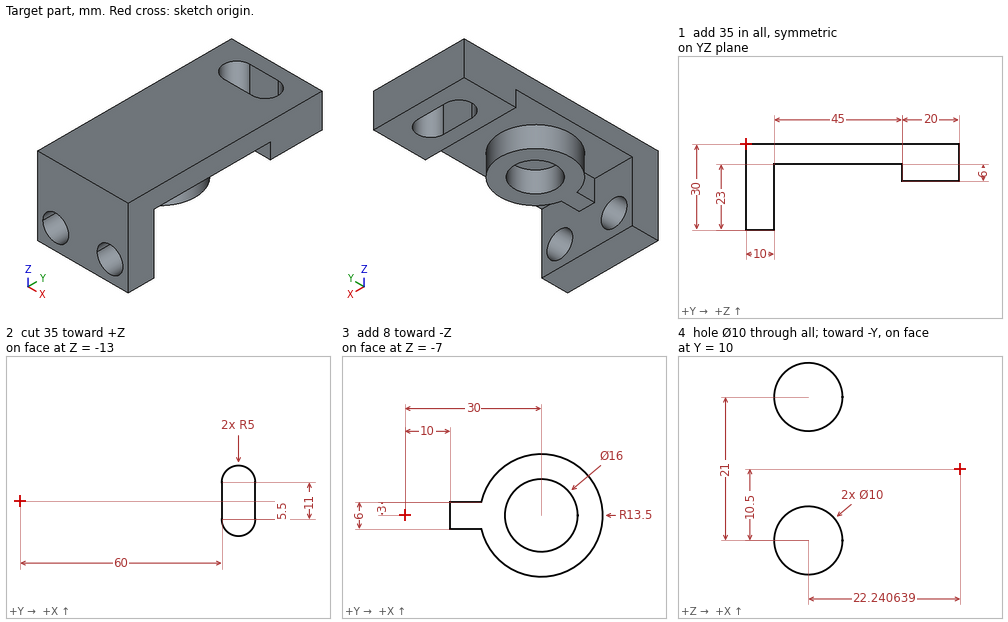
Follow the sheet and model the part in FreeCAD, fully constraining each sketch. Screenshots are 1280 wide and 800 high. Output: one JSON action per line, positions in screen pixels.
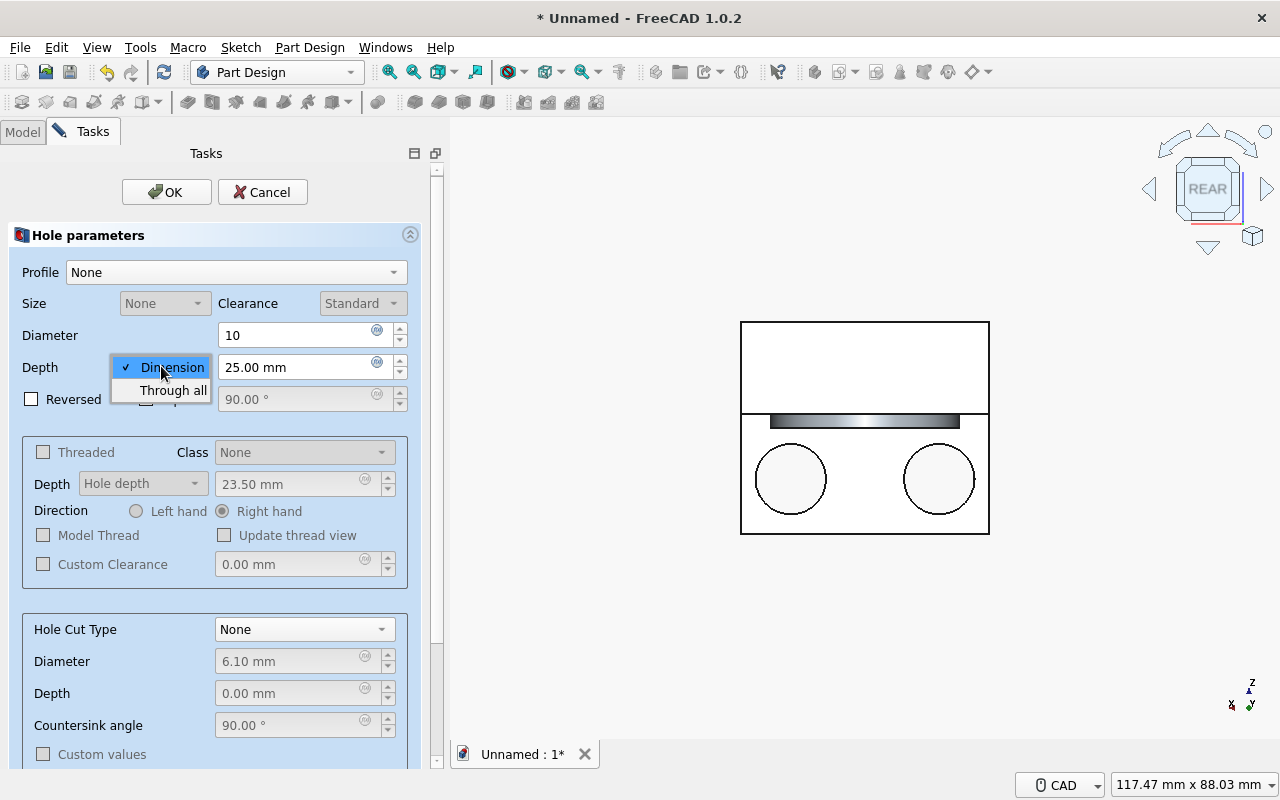
{"action": "left_click", "coordinate": [160, 390]}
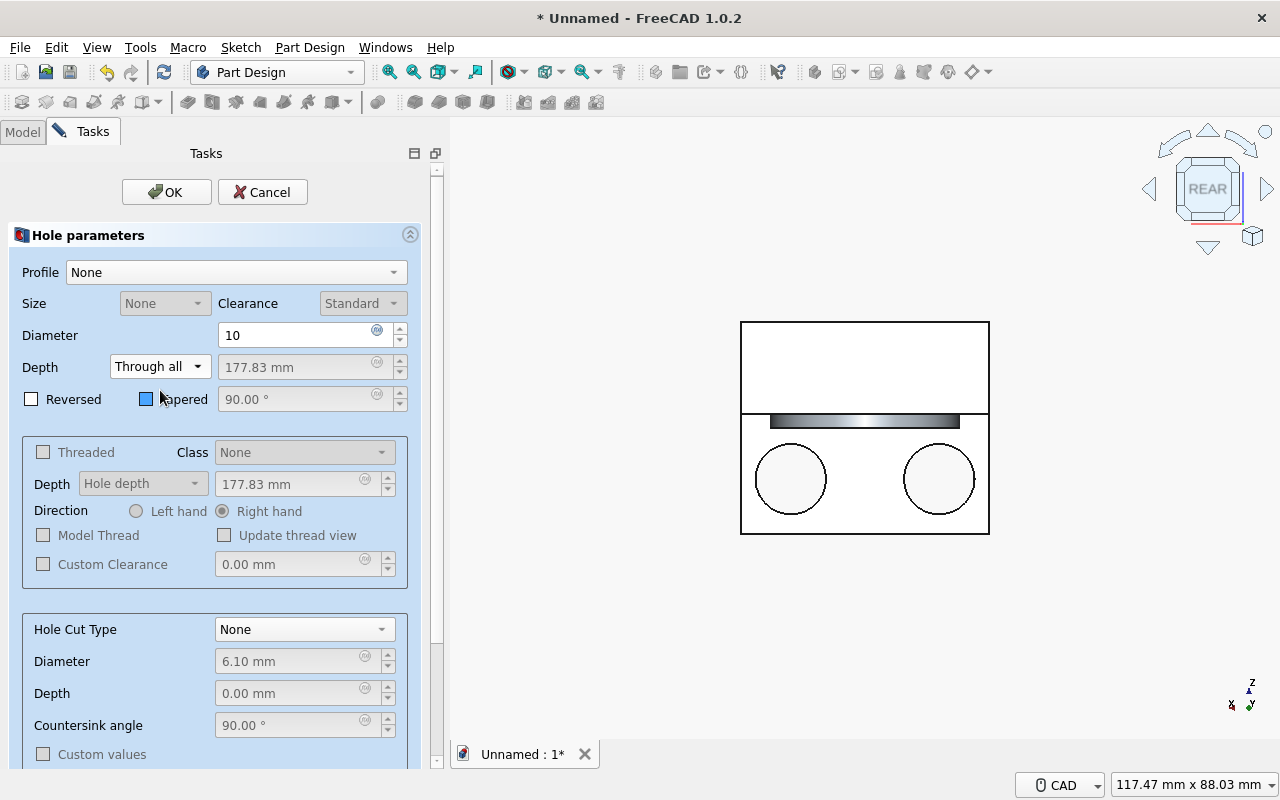
{"action": "left_click", "coordinate": [167, 192]}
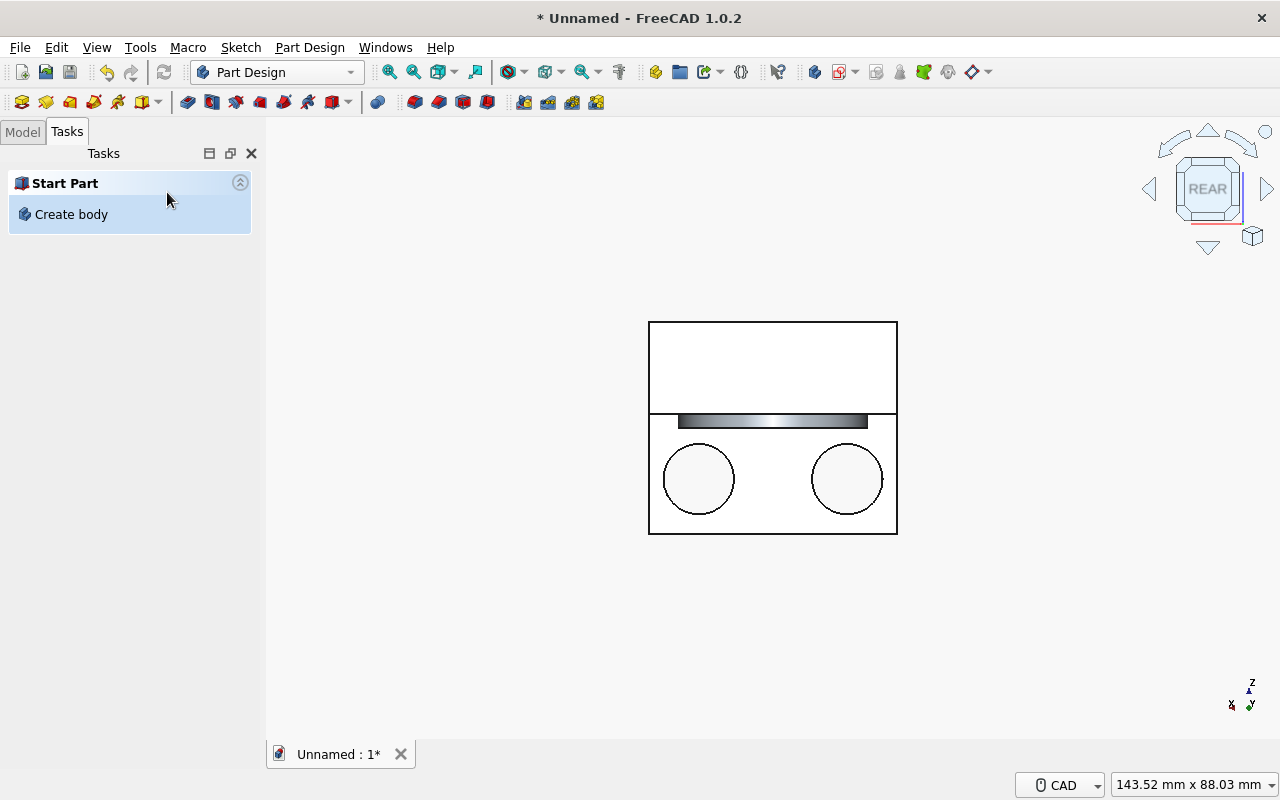
{"action": "key", "text": "0"}